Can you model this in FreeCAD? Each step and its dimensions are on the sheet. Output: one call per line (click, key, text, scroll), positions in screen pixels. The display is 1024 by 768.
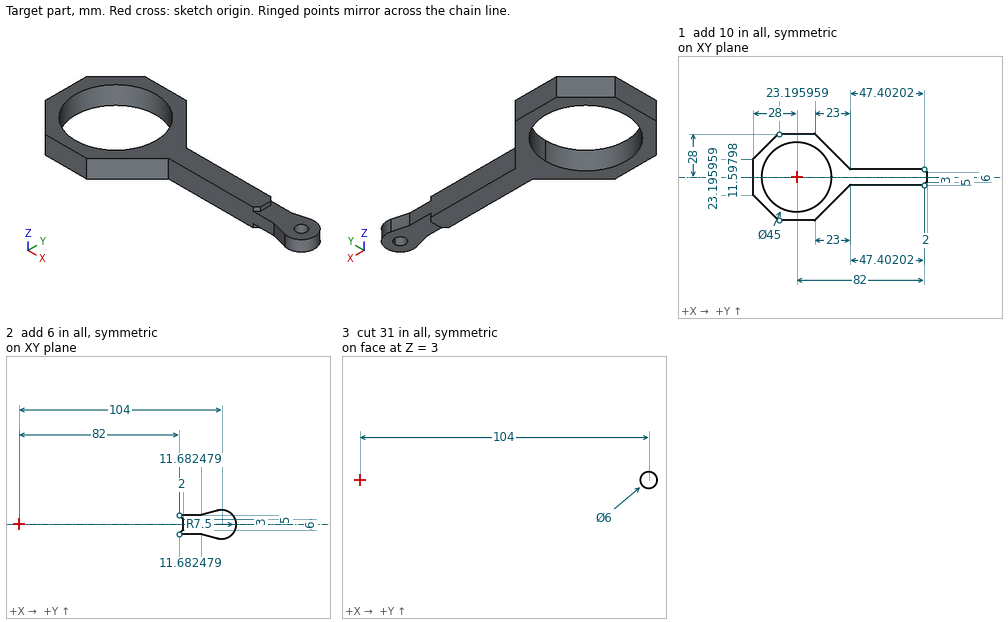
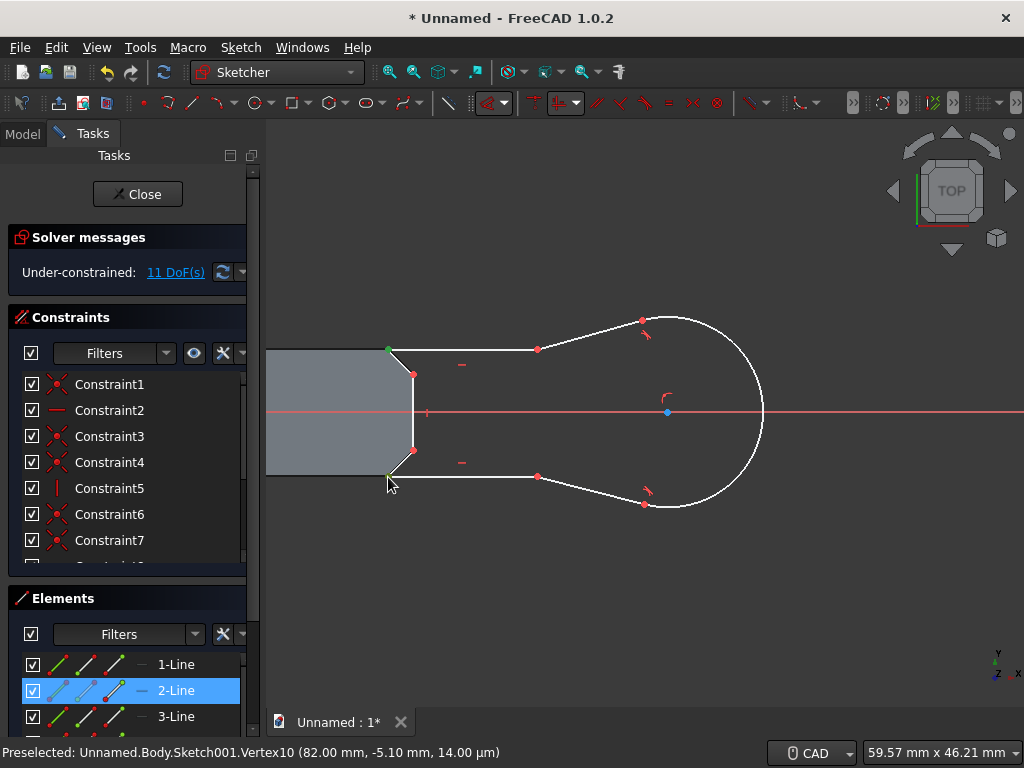
click(334, 412)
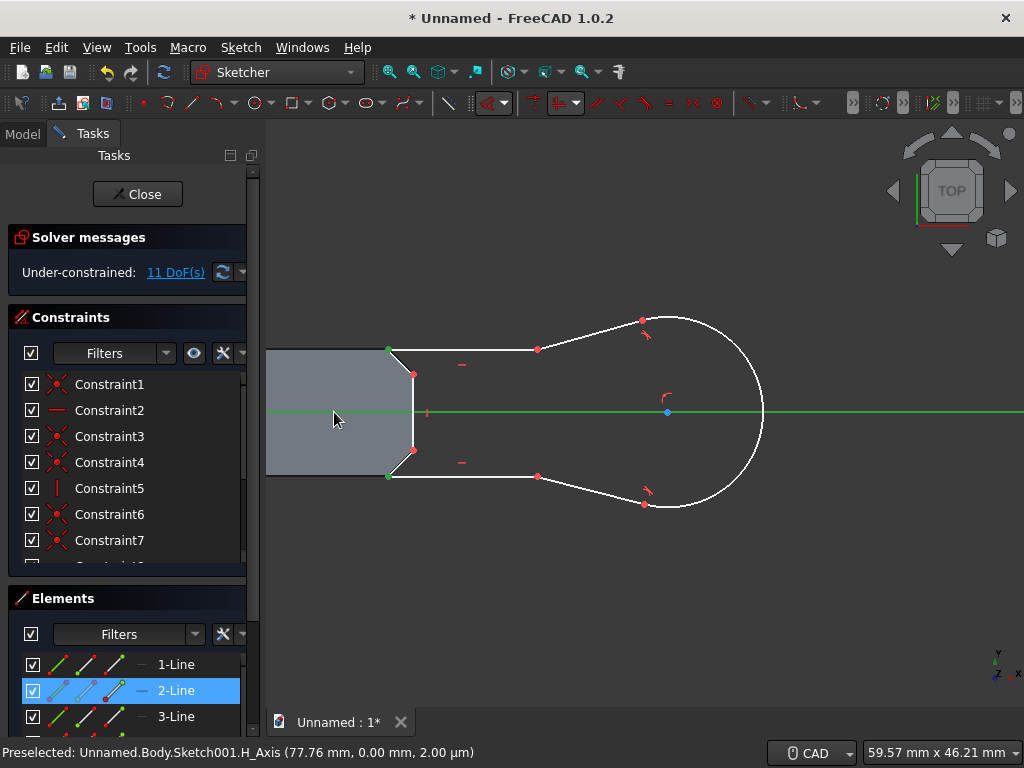
click(694, 104)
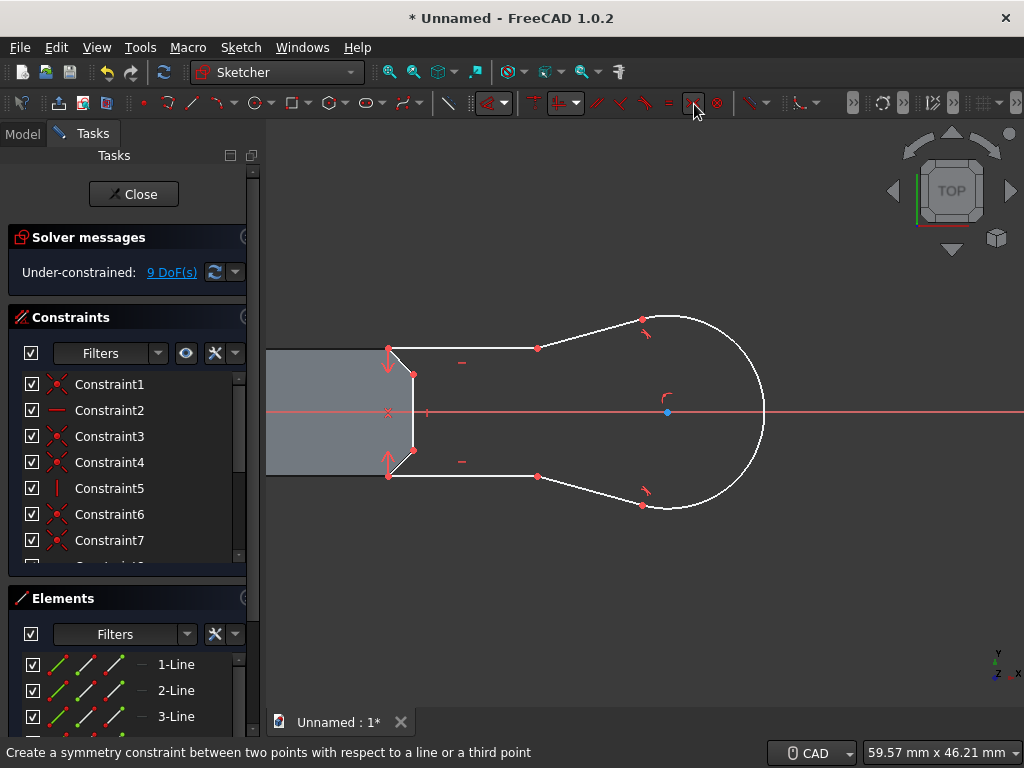
click(739, 477)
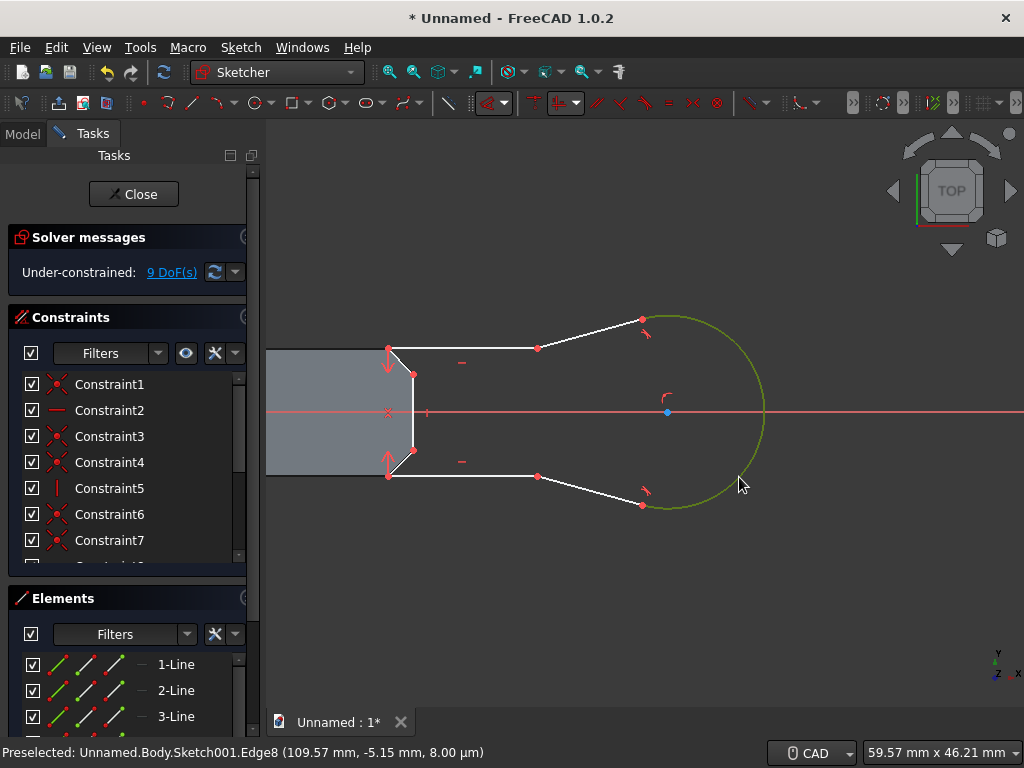
click(506, 104)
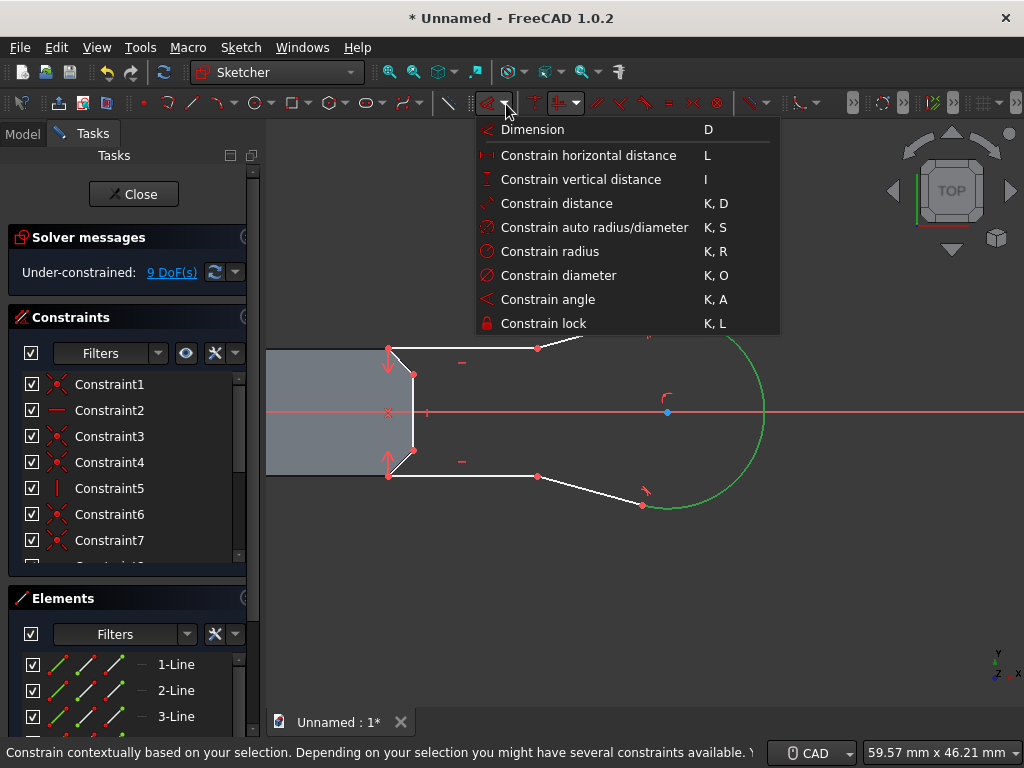
click(628, 251)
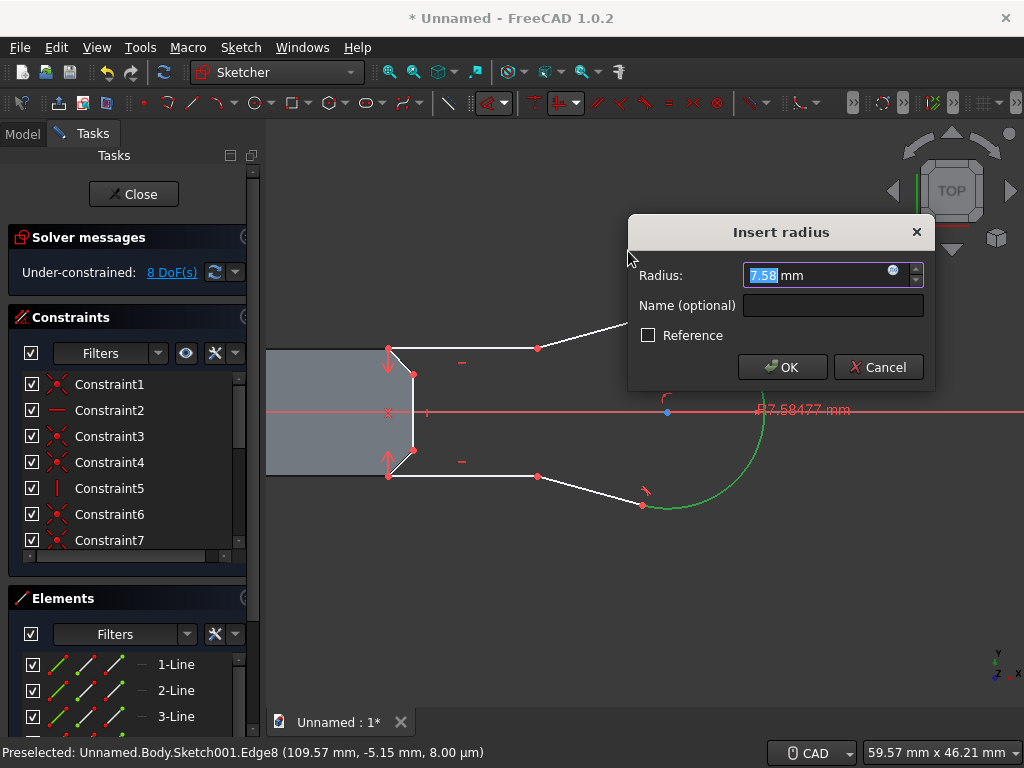
text(7.5)
key(Return)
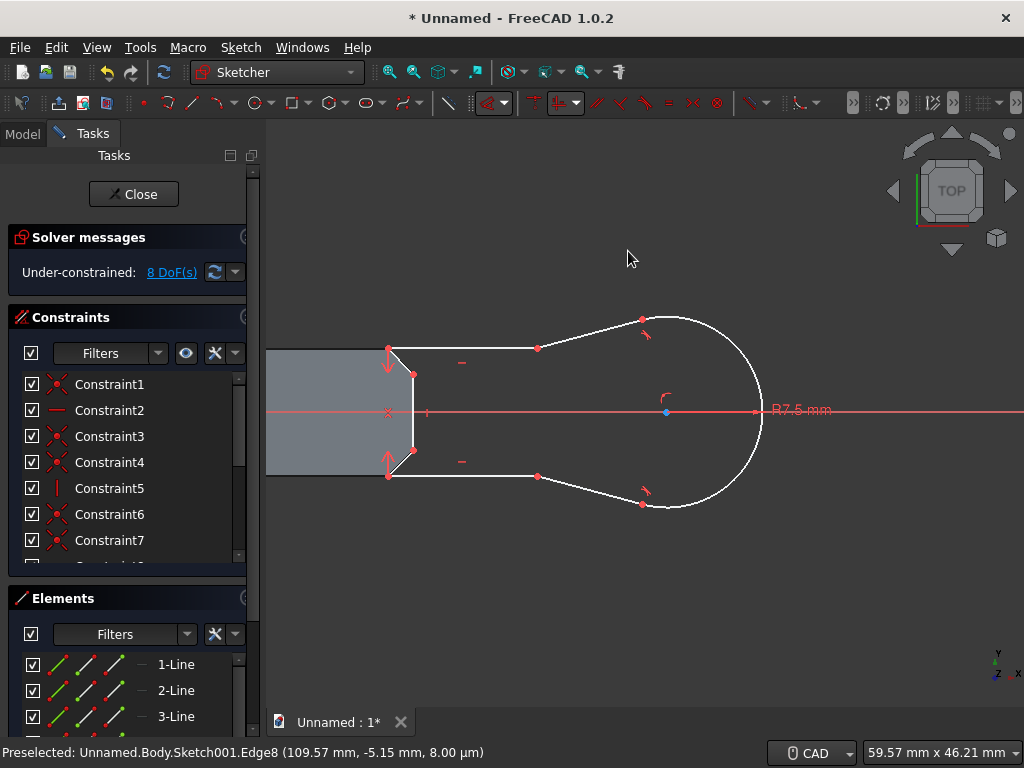
click(413, 398)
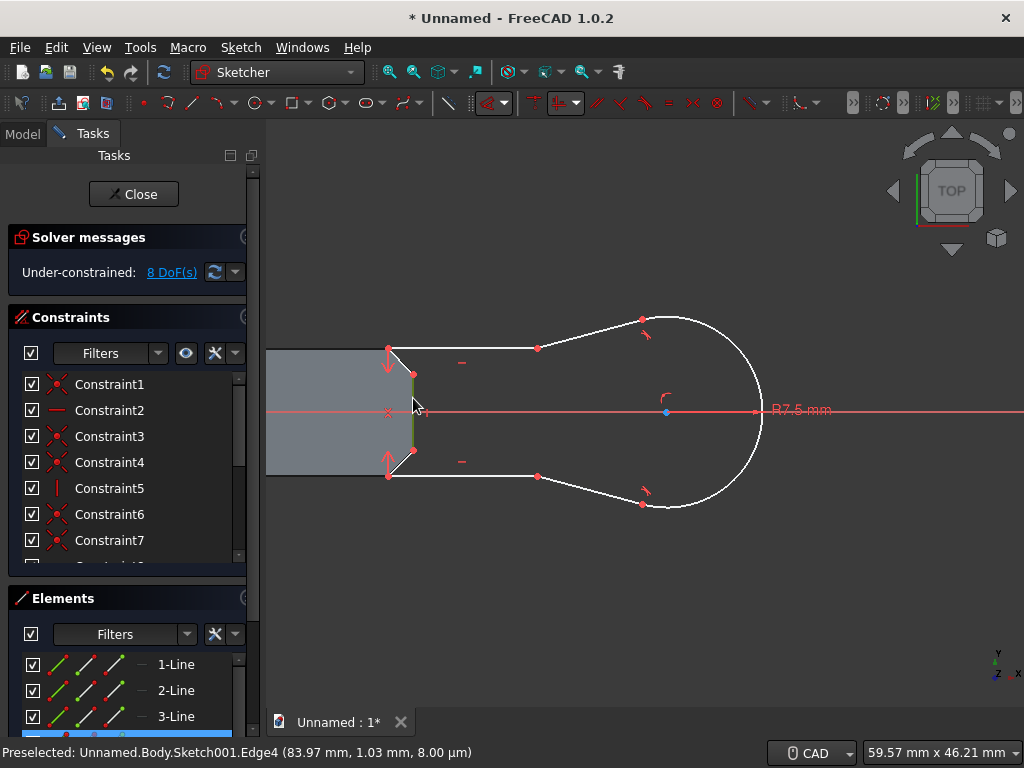
key(i)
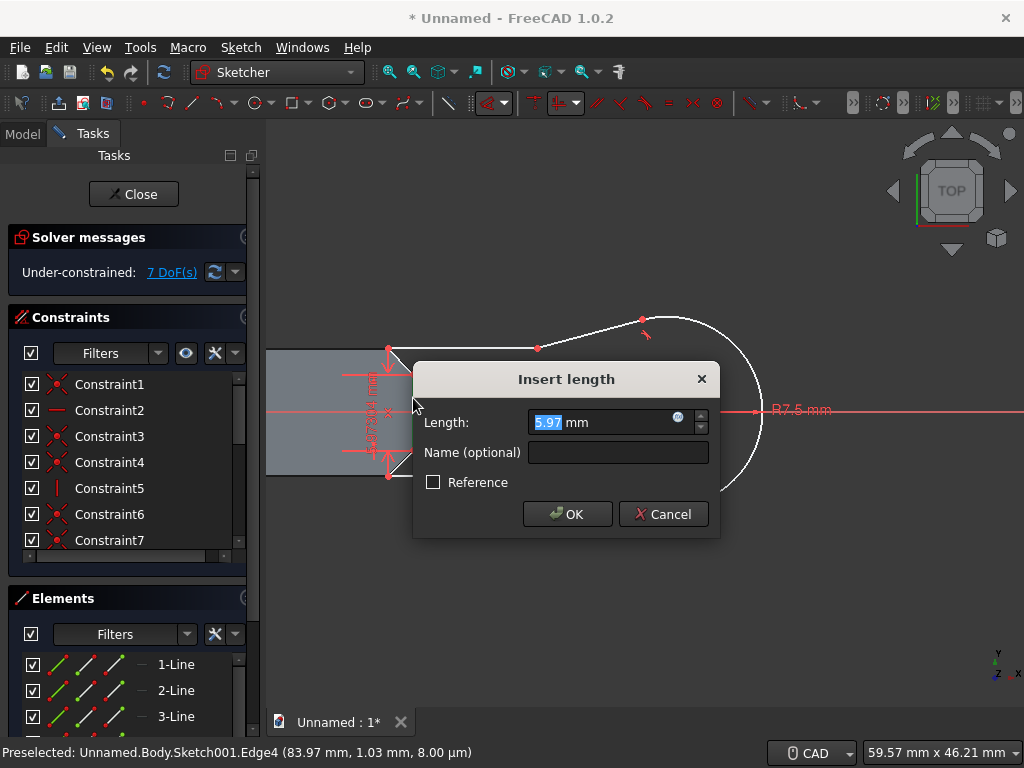
text(6)
key(Return)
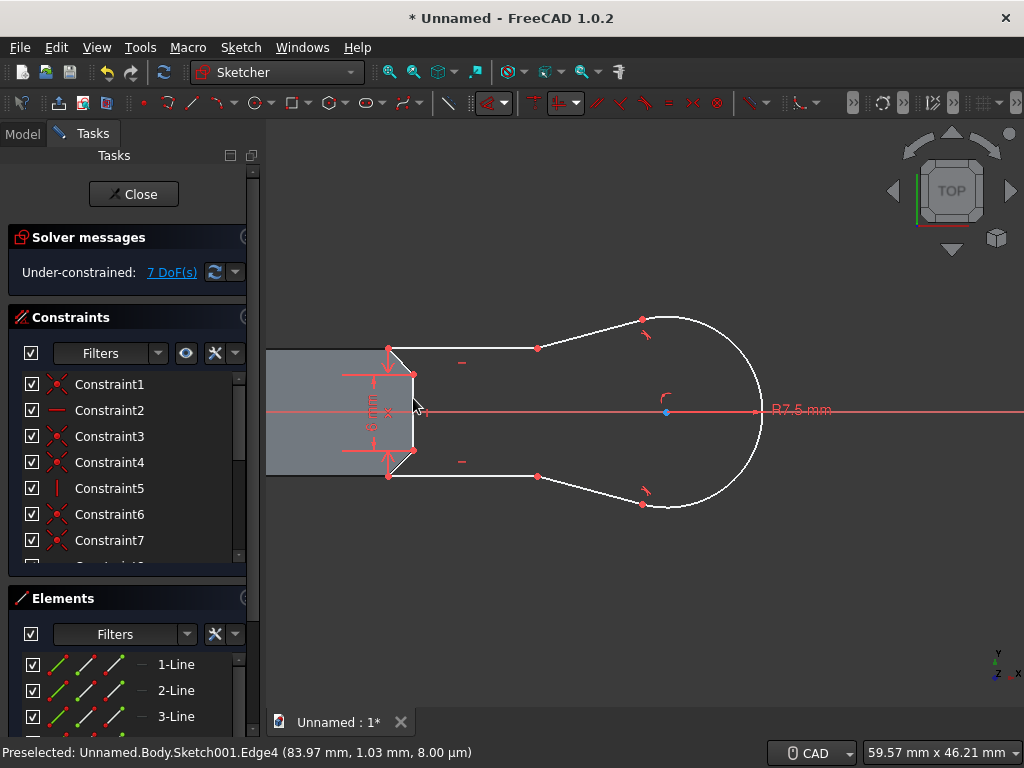
click(537, 348)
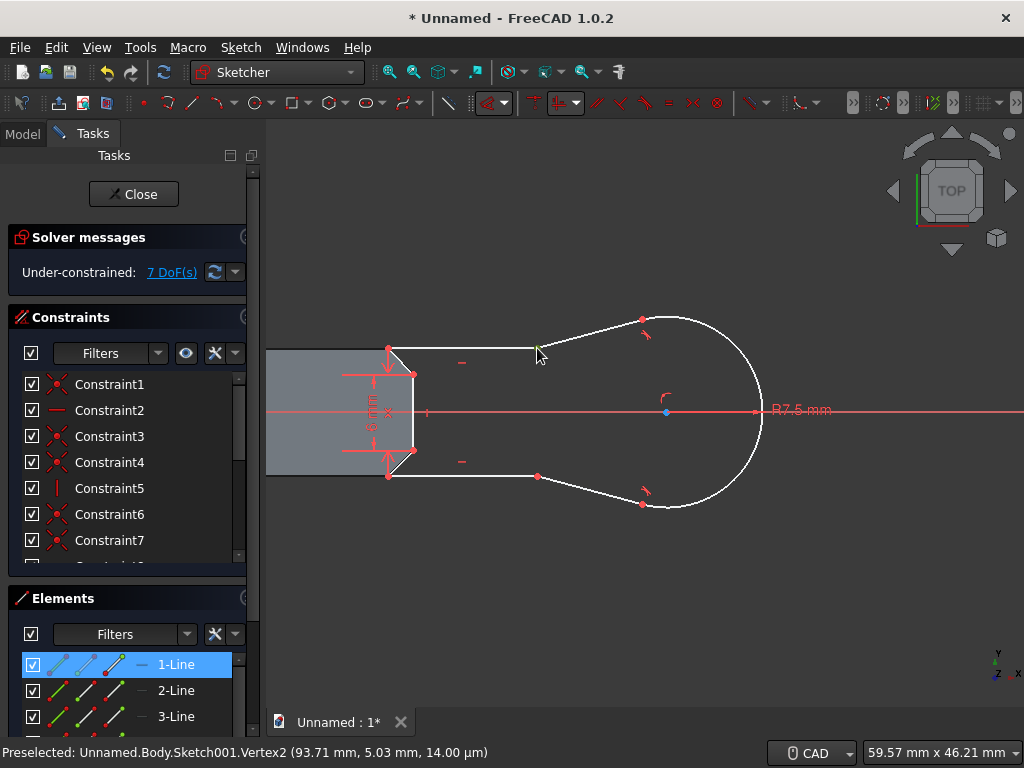
click(506, 104)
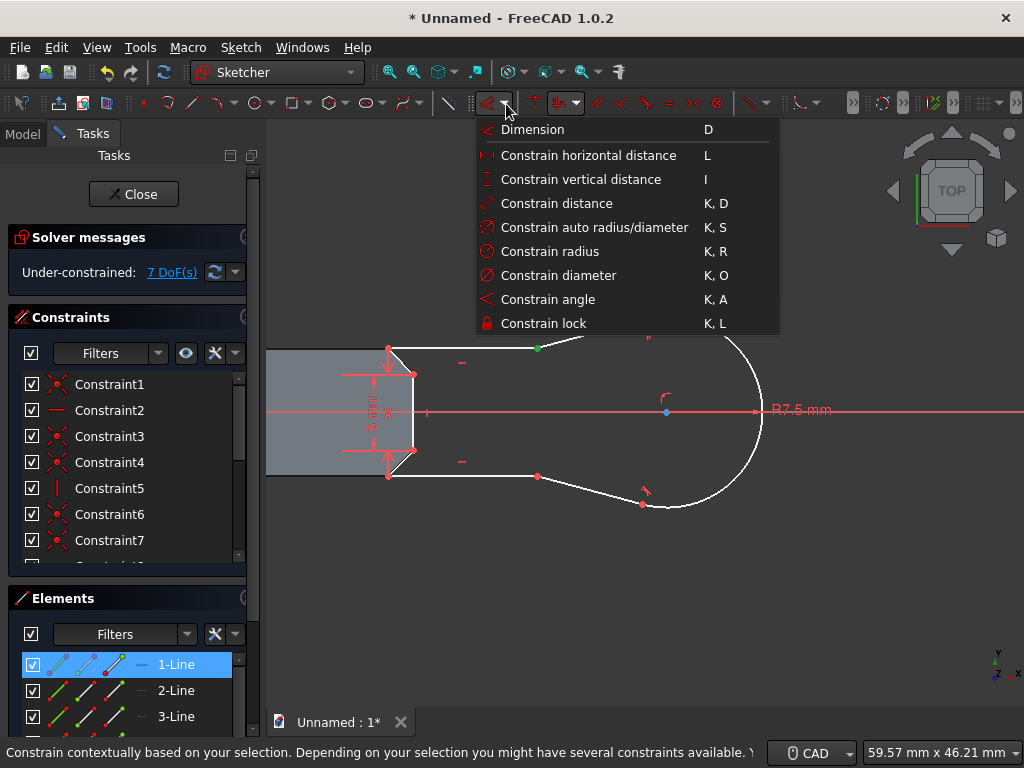
click(628, 179)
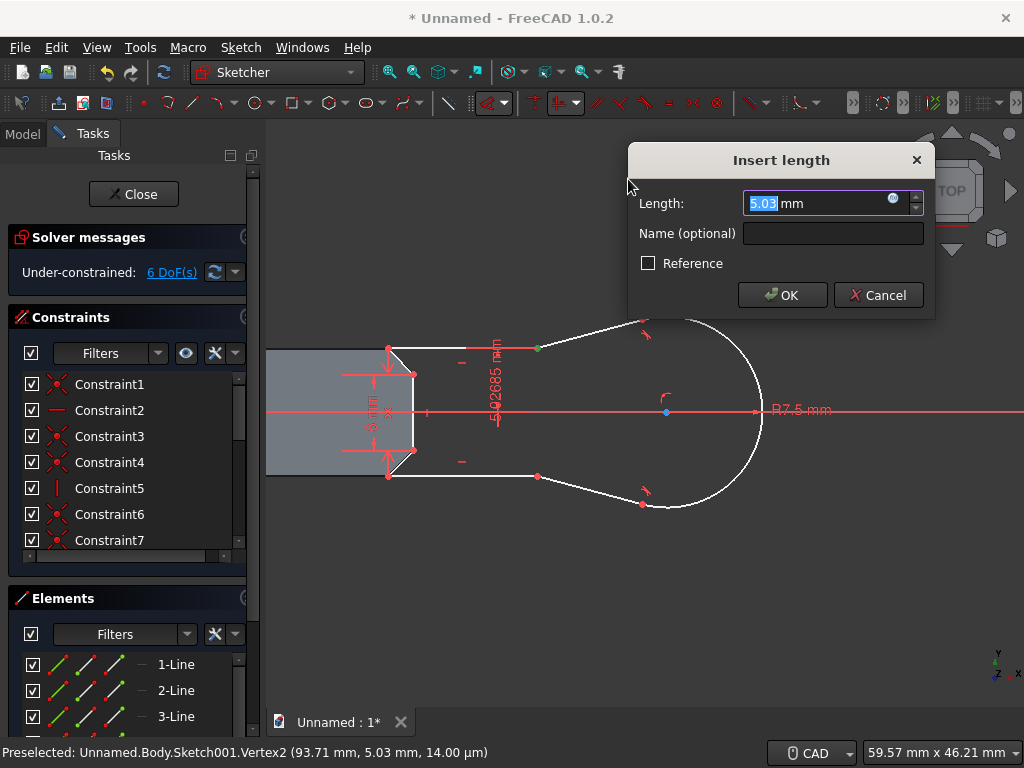
text(5)
key(Return)